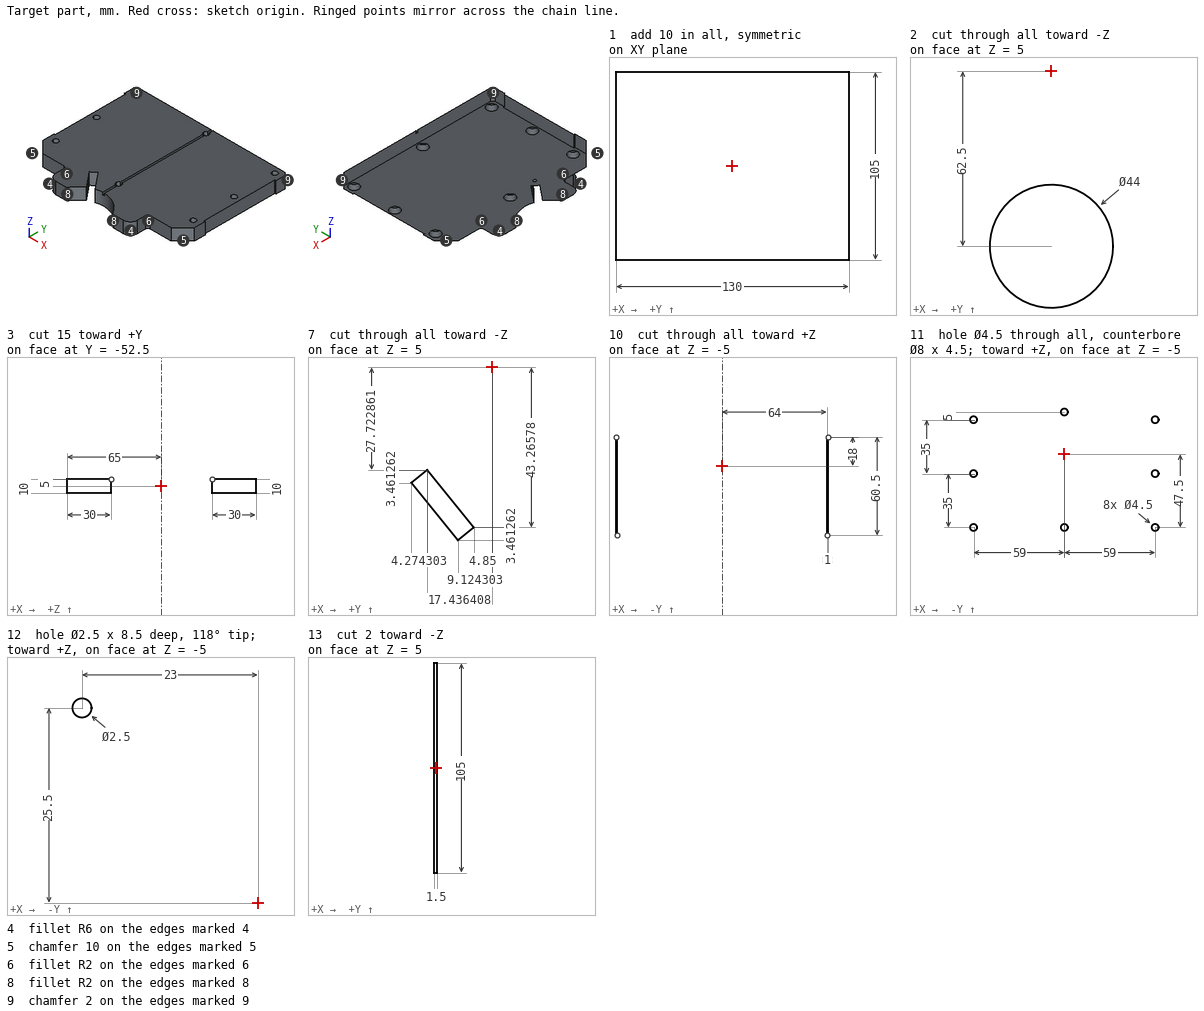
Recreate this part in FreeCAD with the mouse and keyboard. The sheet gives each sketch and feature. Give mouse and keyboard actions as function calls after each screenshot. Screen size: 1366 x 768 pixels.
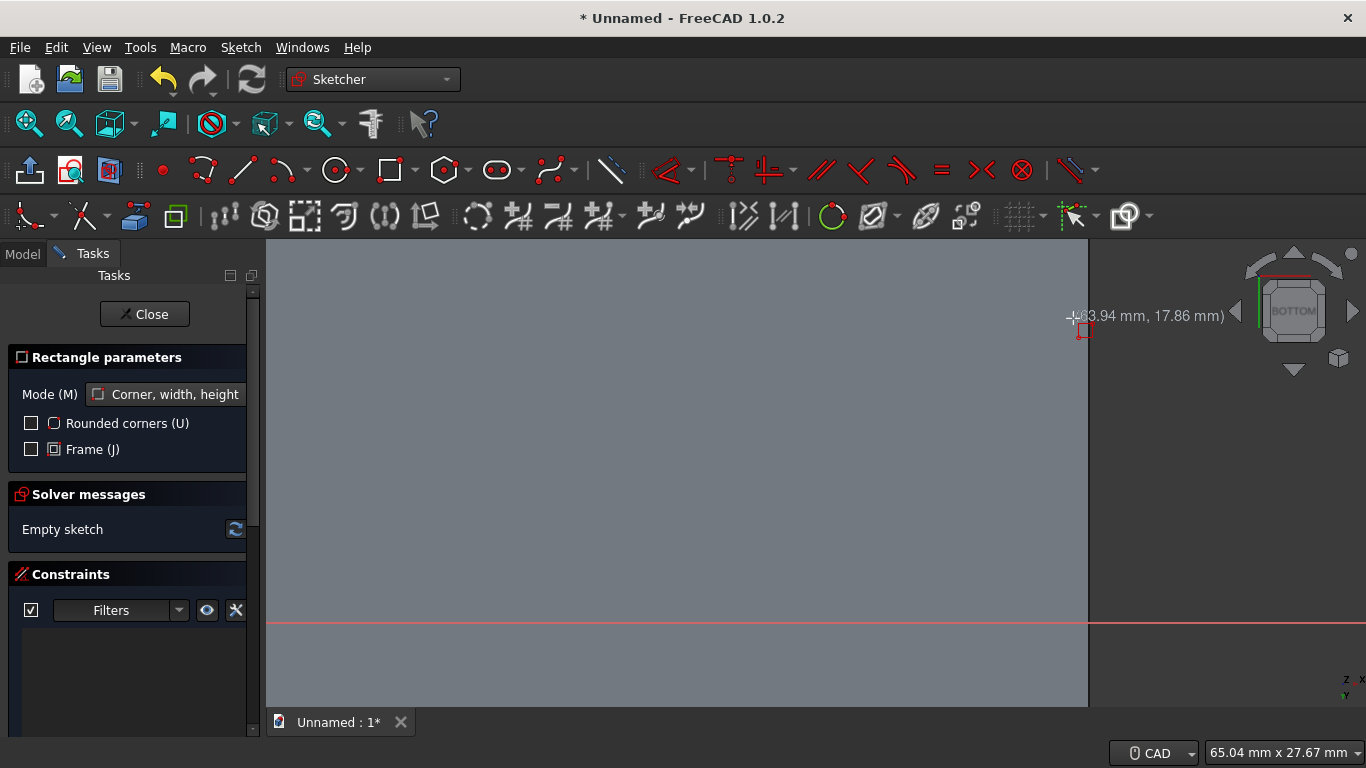
click(1072, 319)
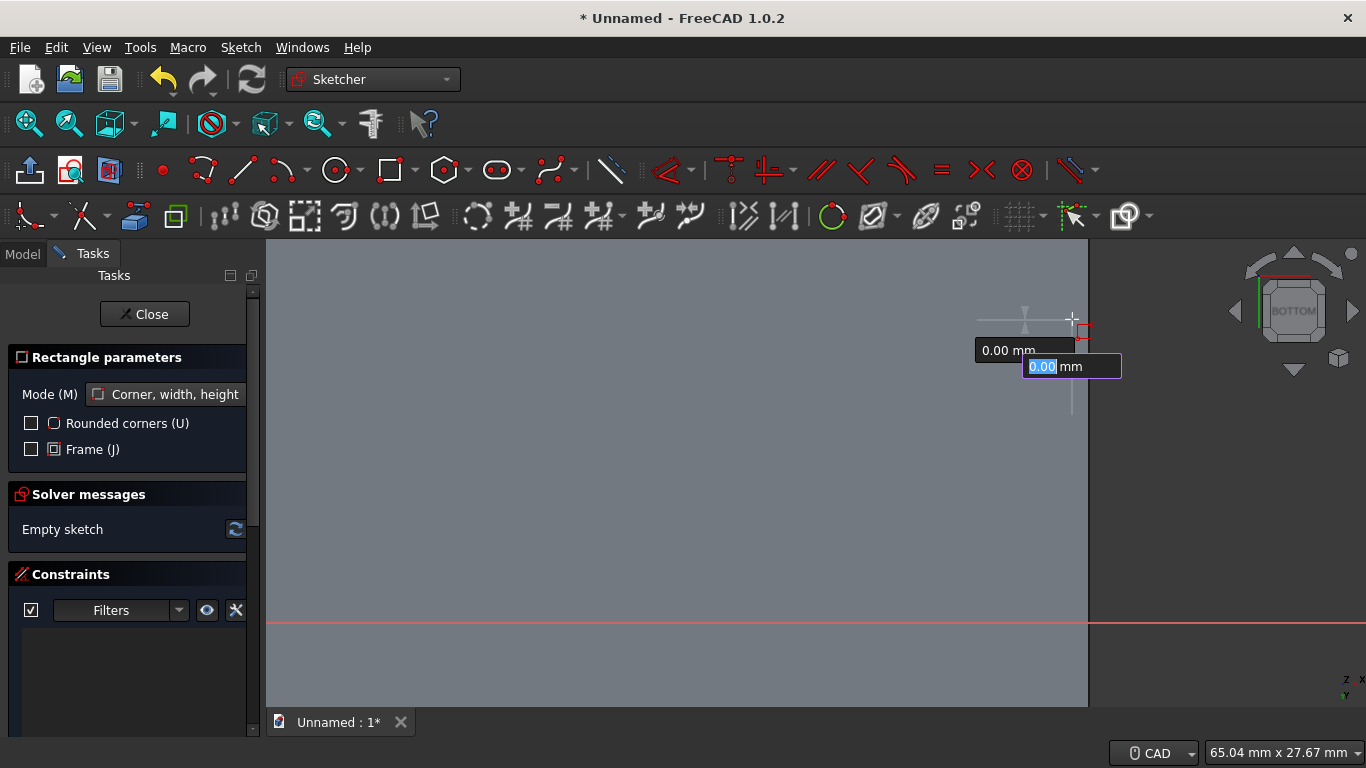
scroll(1074, 319, down, 6)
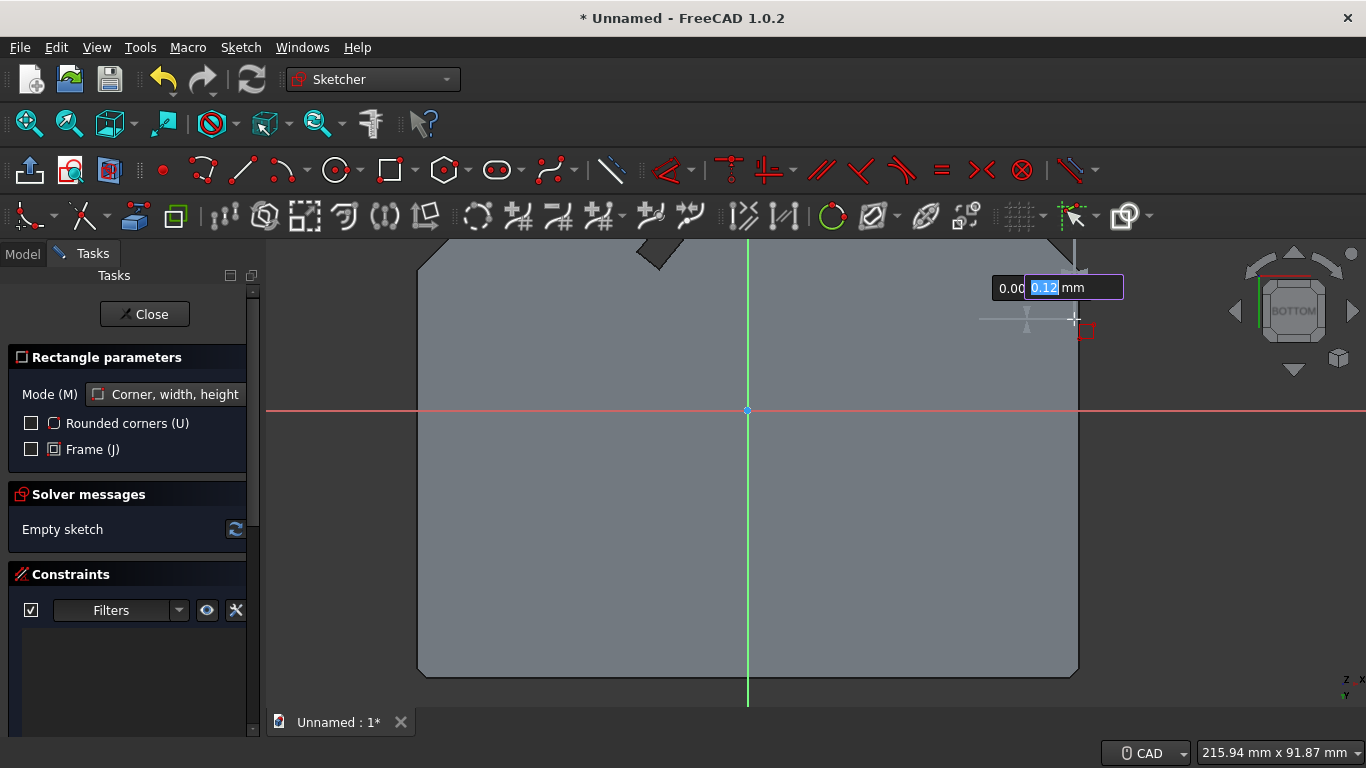
click(1079, 627)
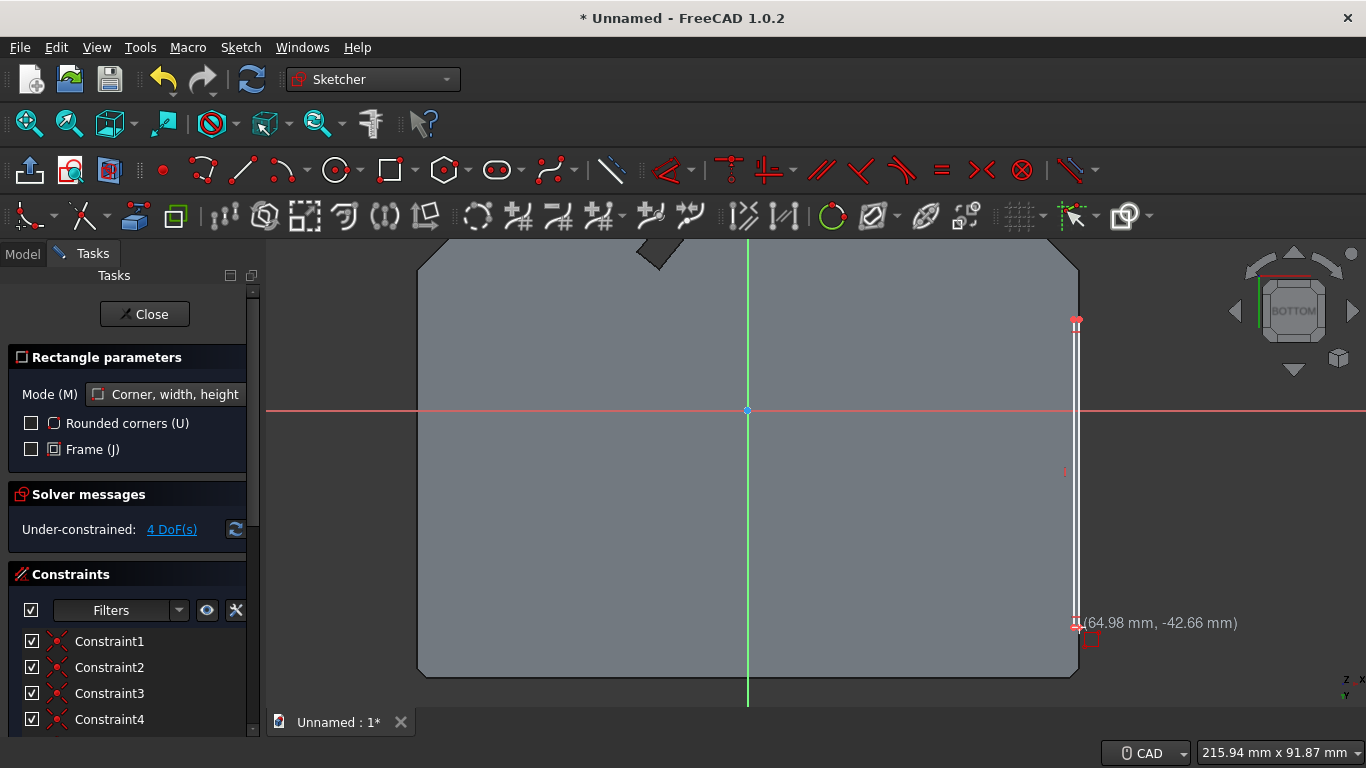
scroll(417, 319, up, 6)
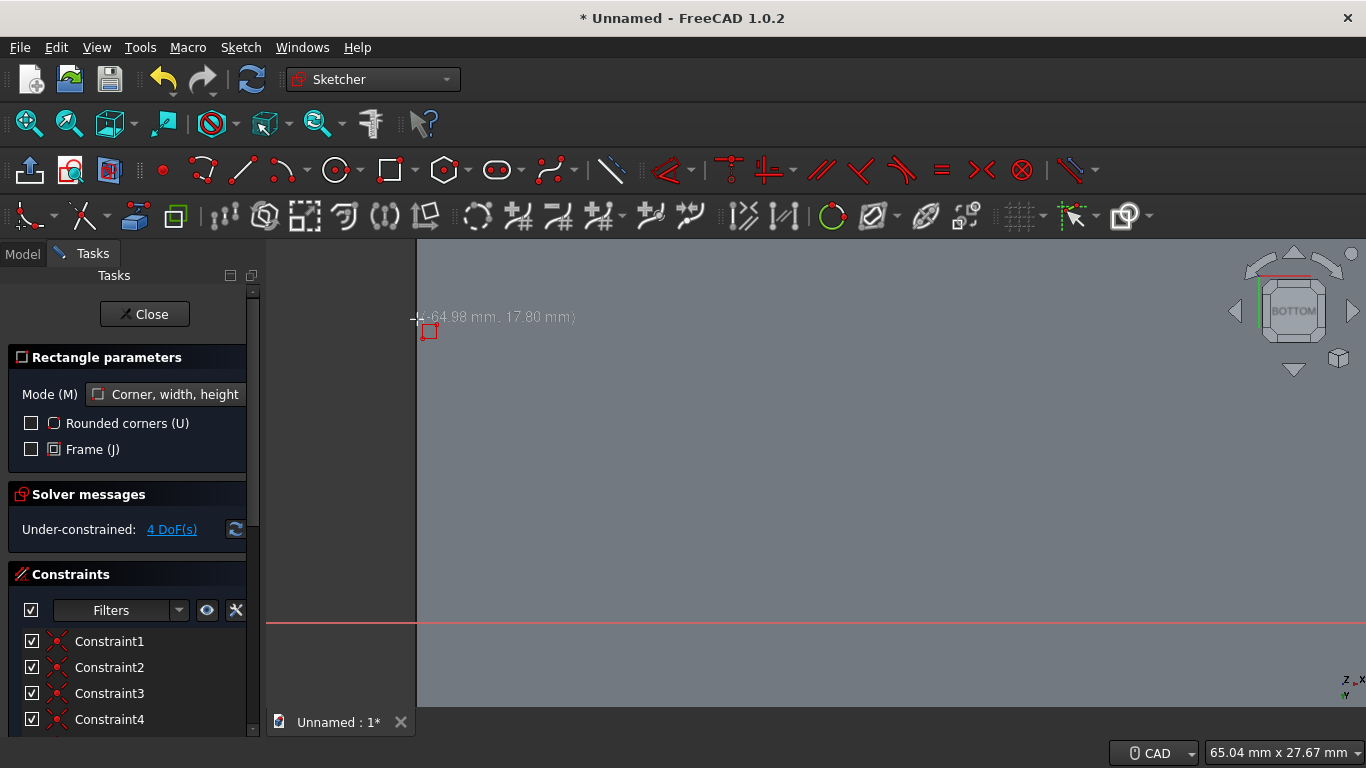
click(416, 319)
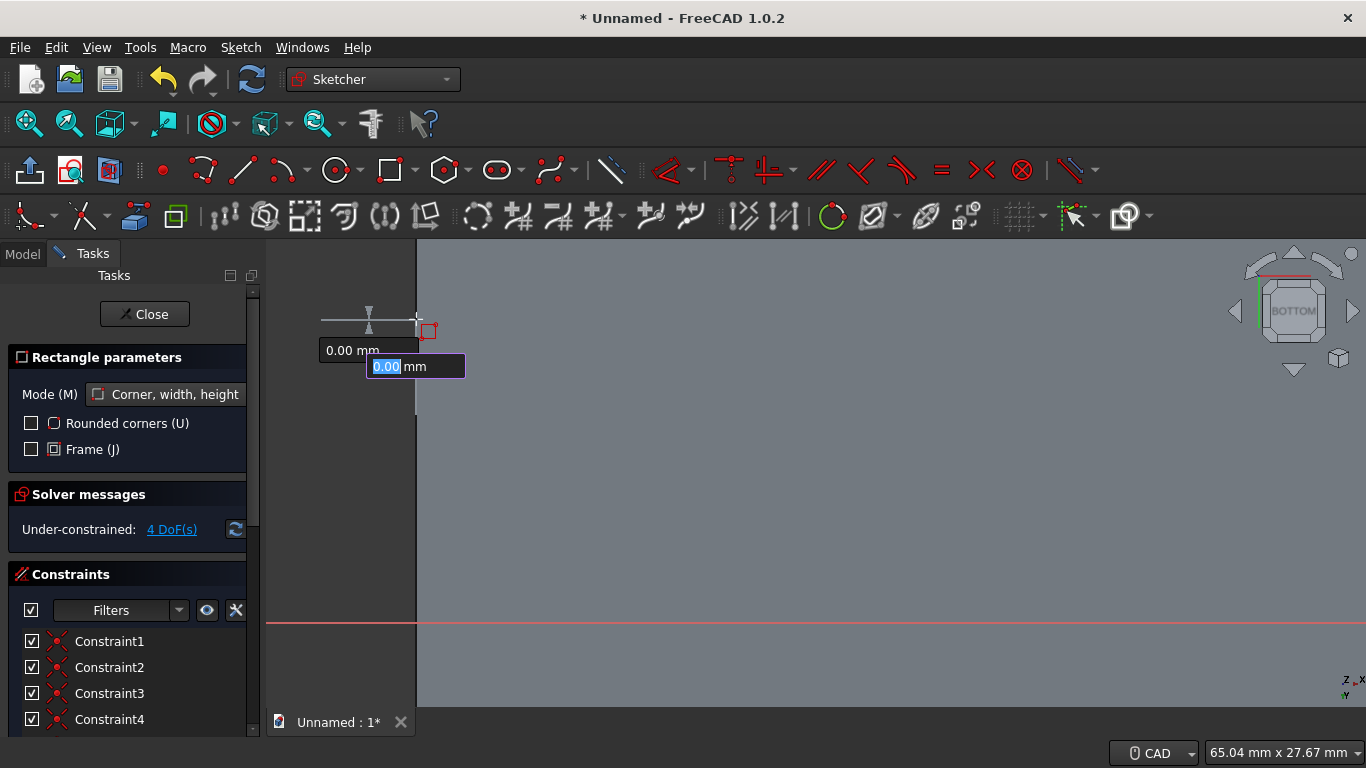
scroll(416, 319, down, 6)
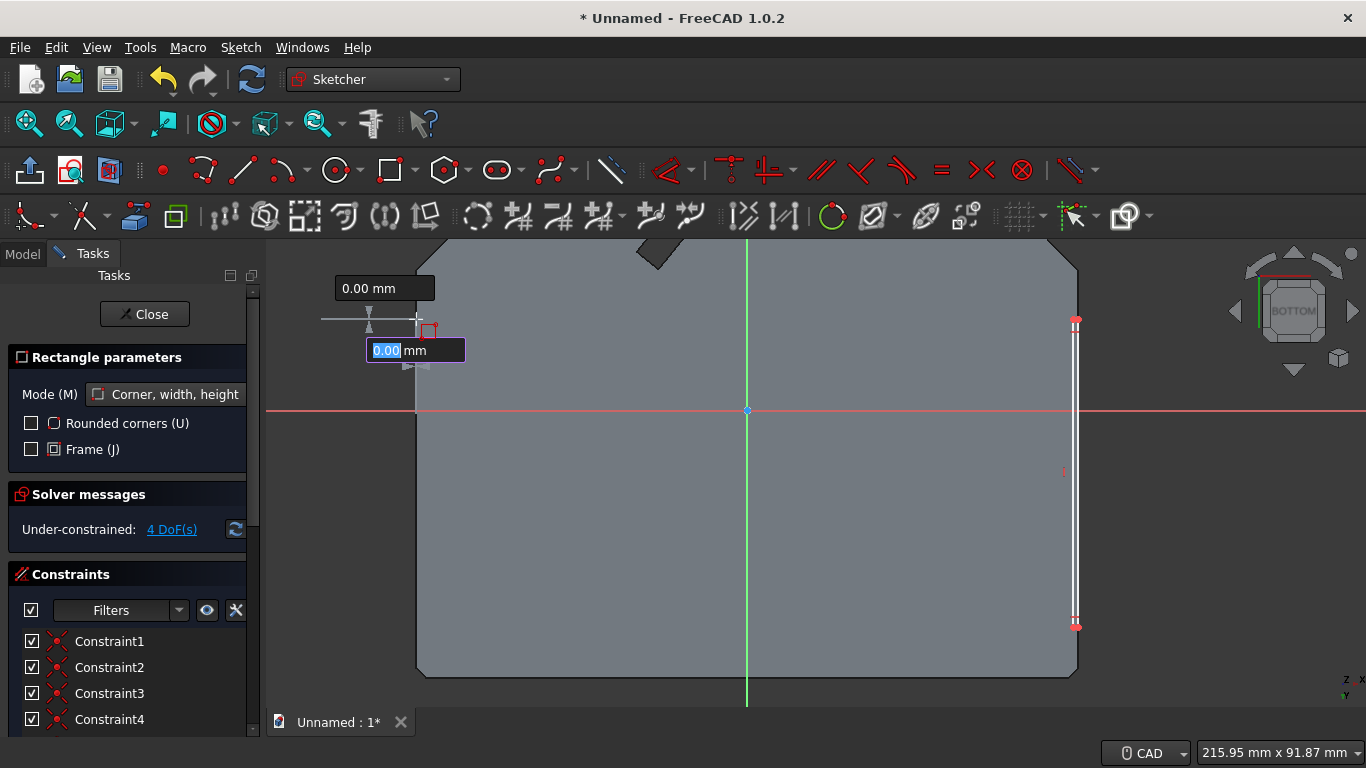
click(421, 627)
key(Escape)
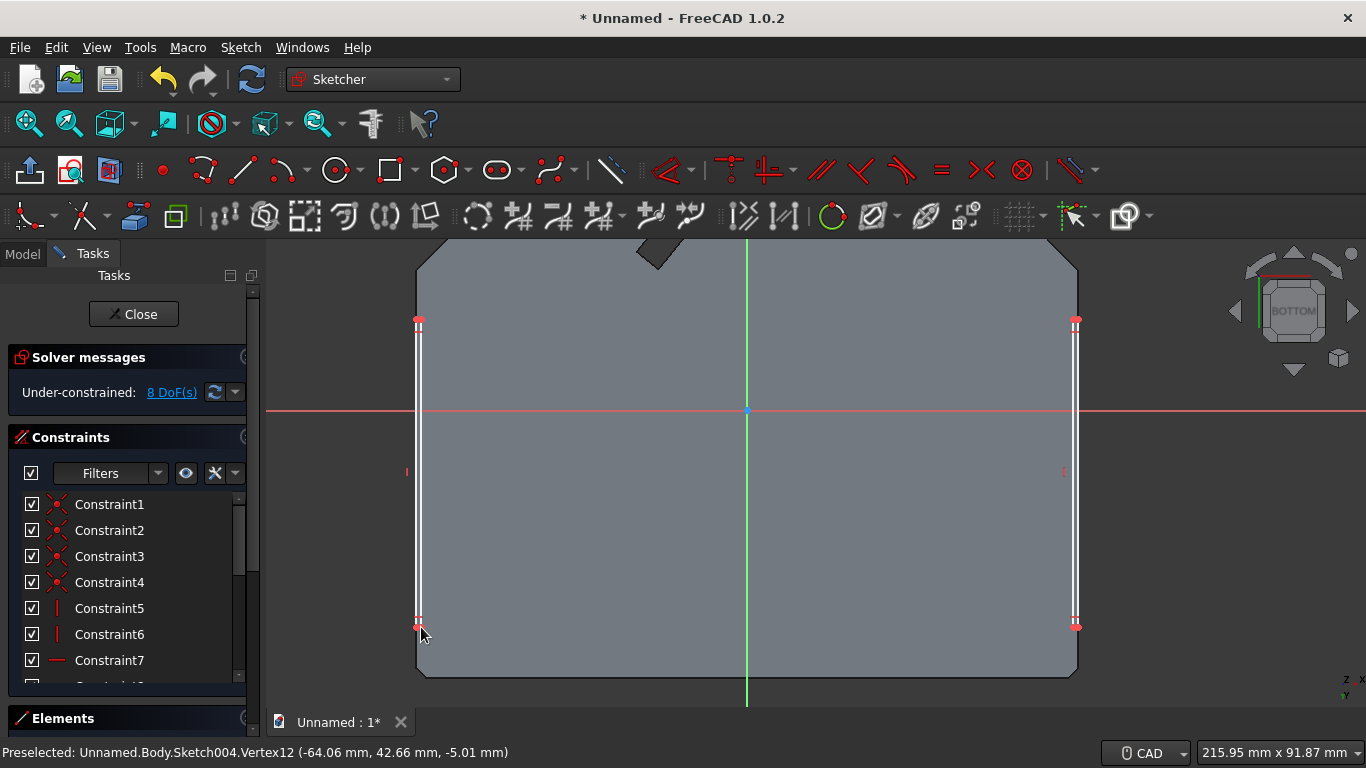
scroll(1078, 319, up, 5)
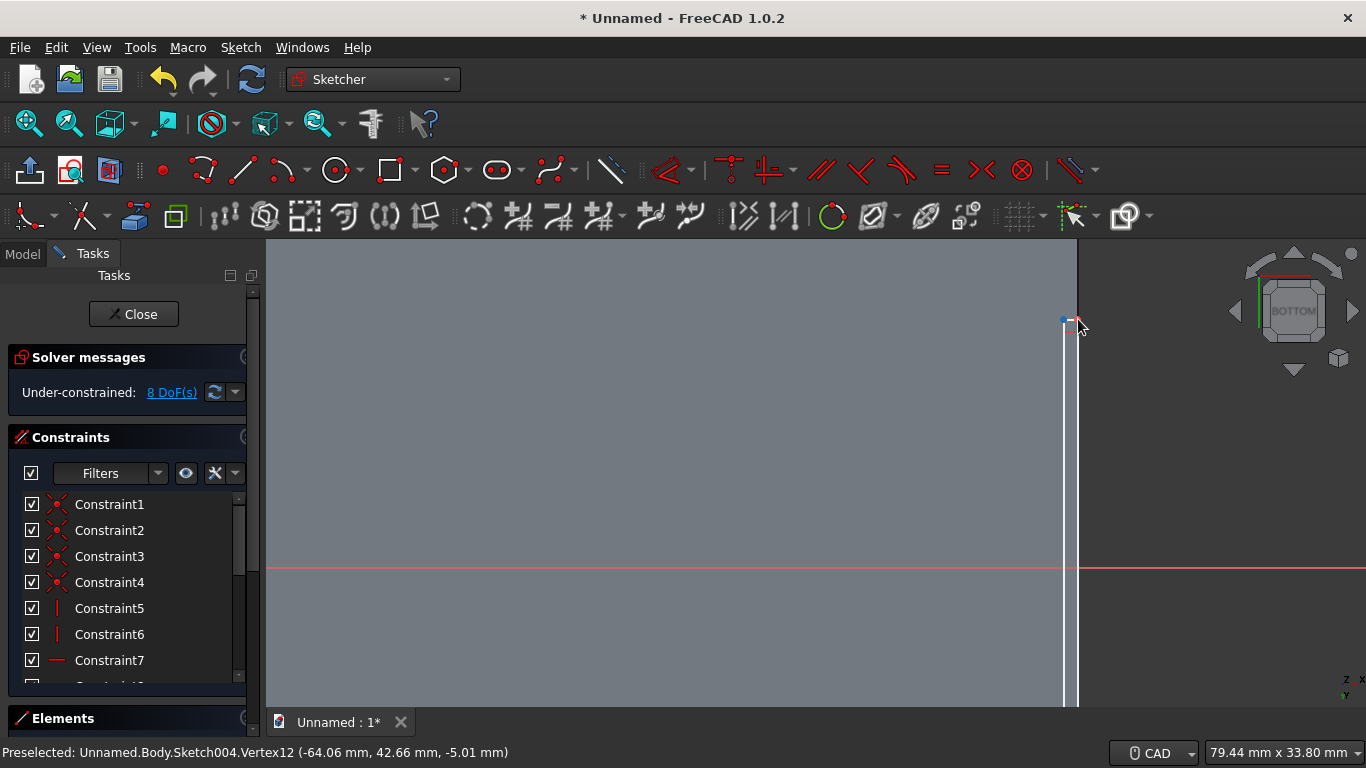
click(1078, 320)